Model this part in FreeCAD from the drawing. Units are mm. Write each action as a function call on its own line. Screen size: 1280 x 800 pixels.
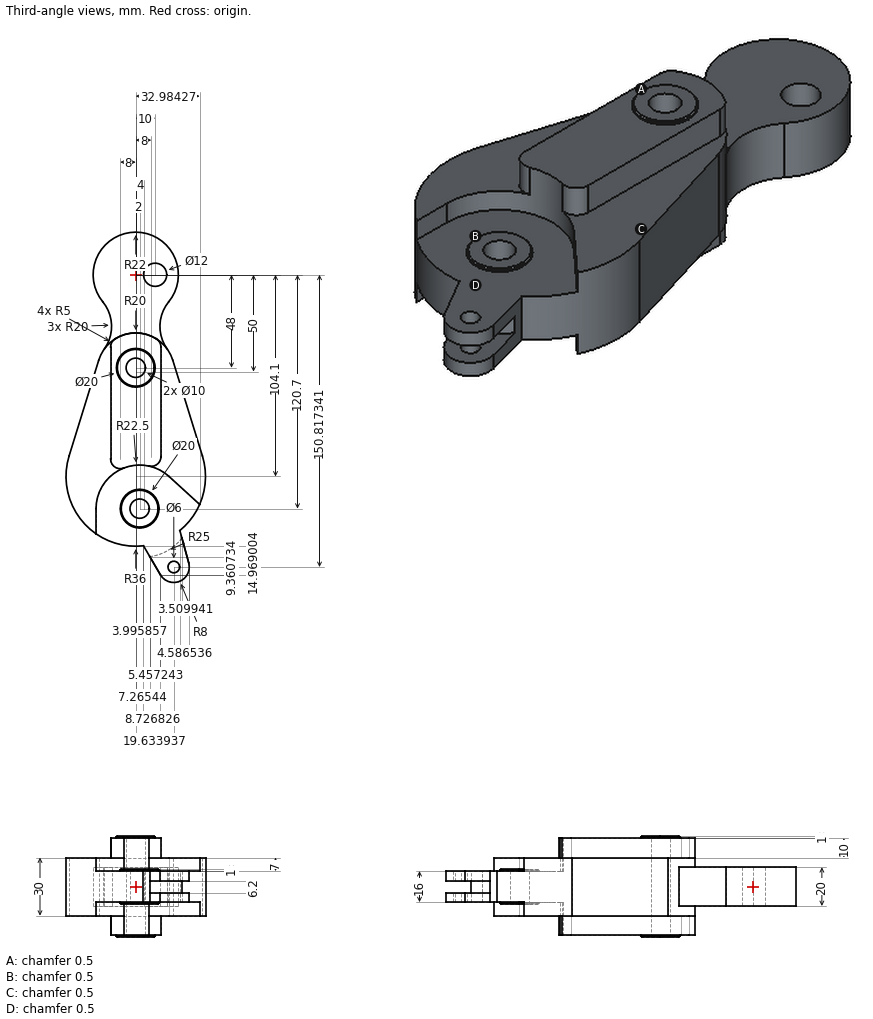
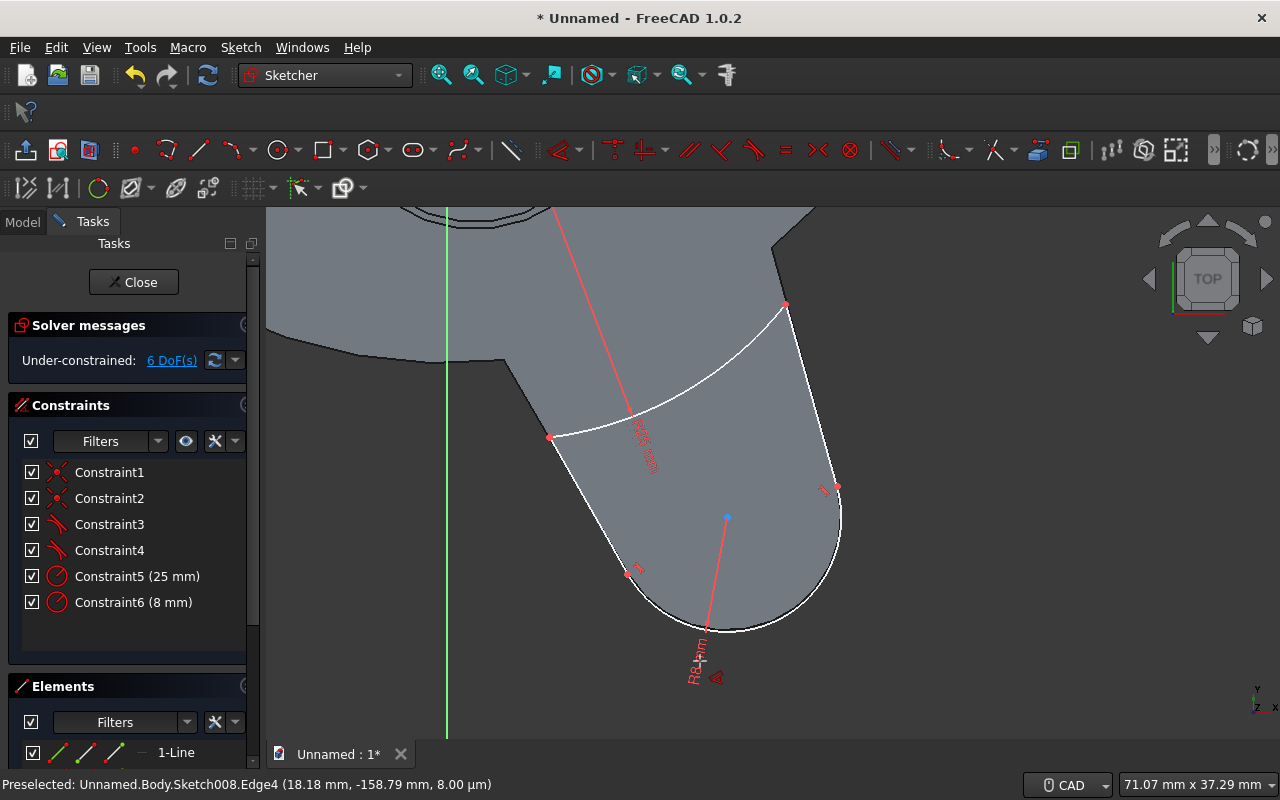
scroll(772, 711, down, 2)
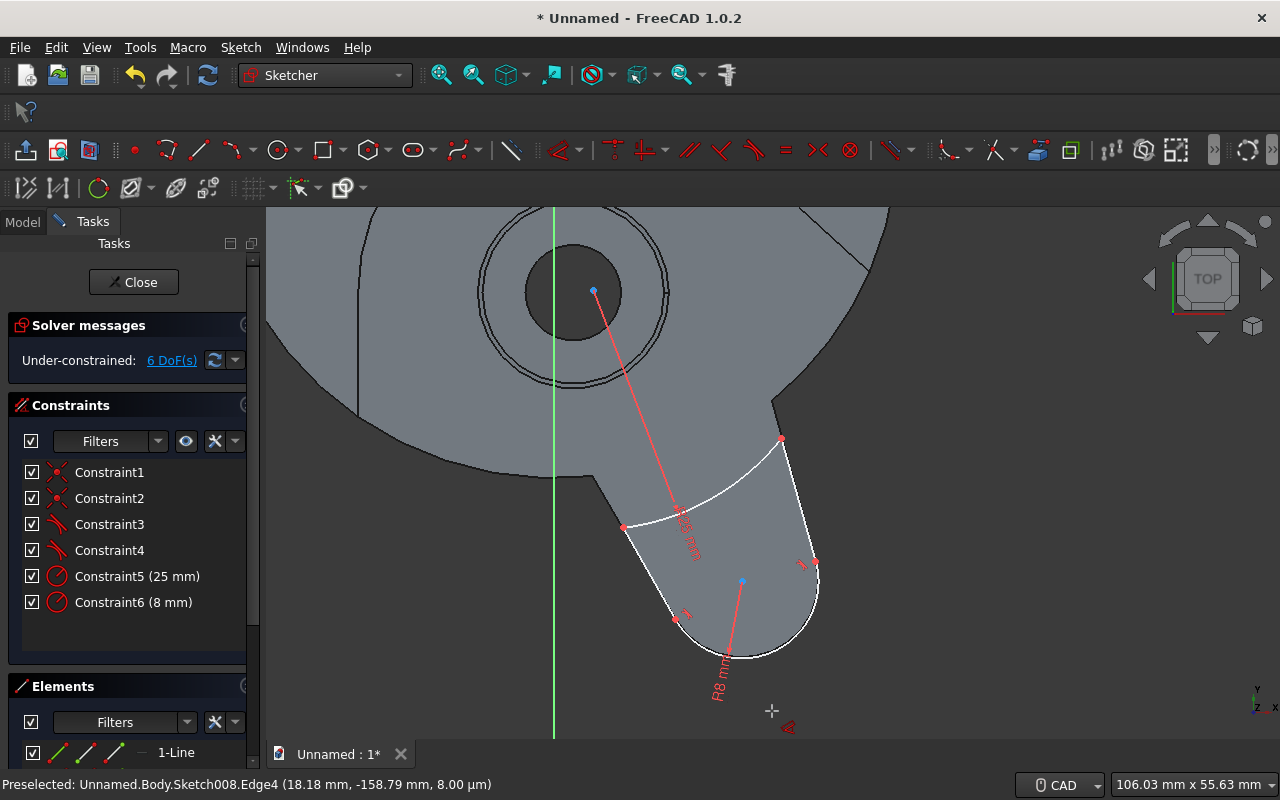
click(594, 291)
click(574, 325)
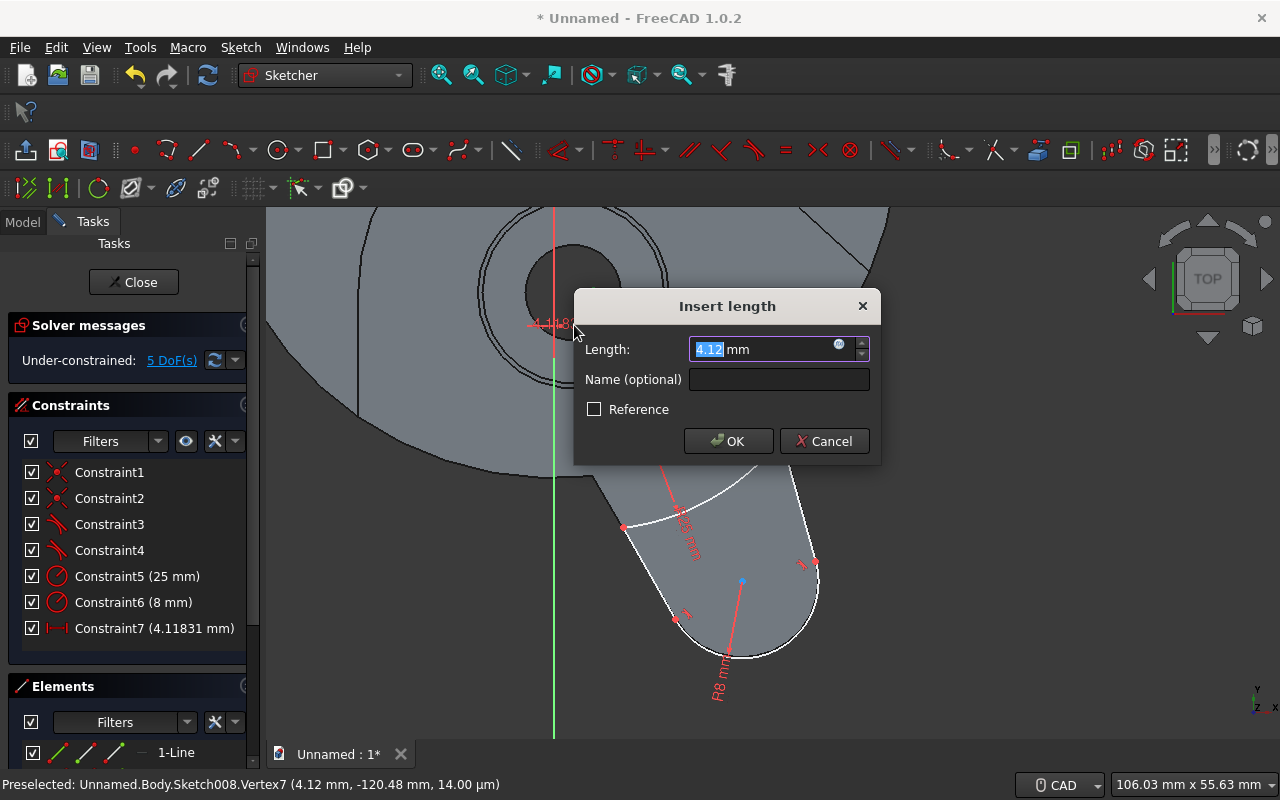
text(4)
key(Return)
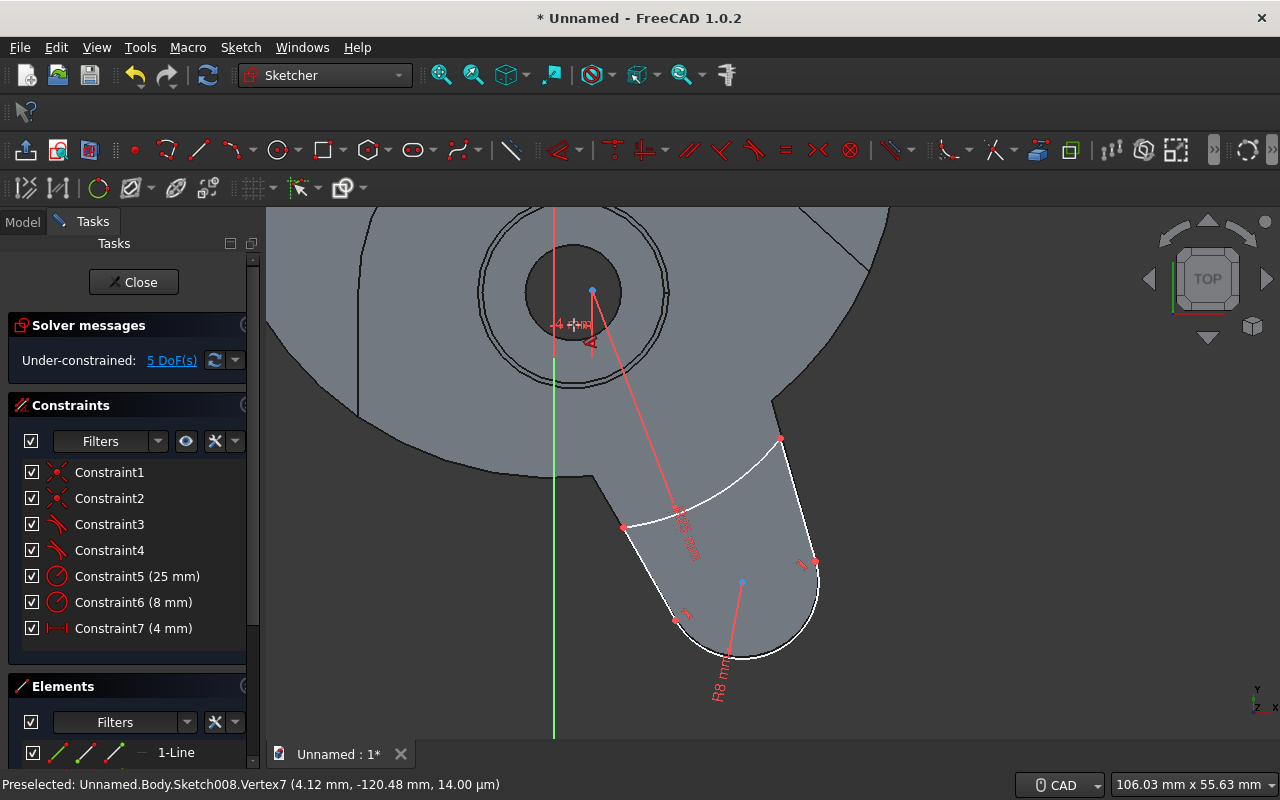
click(592, 291)
click(520, 263)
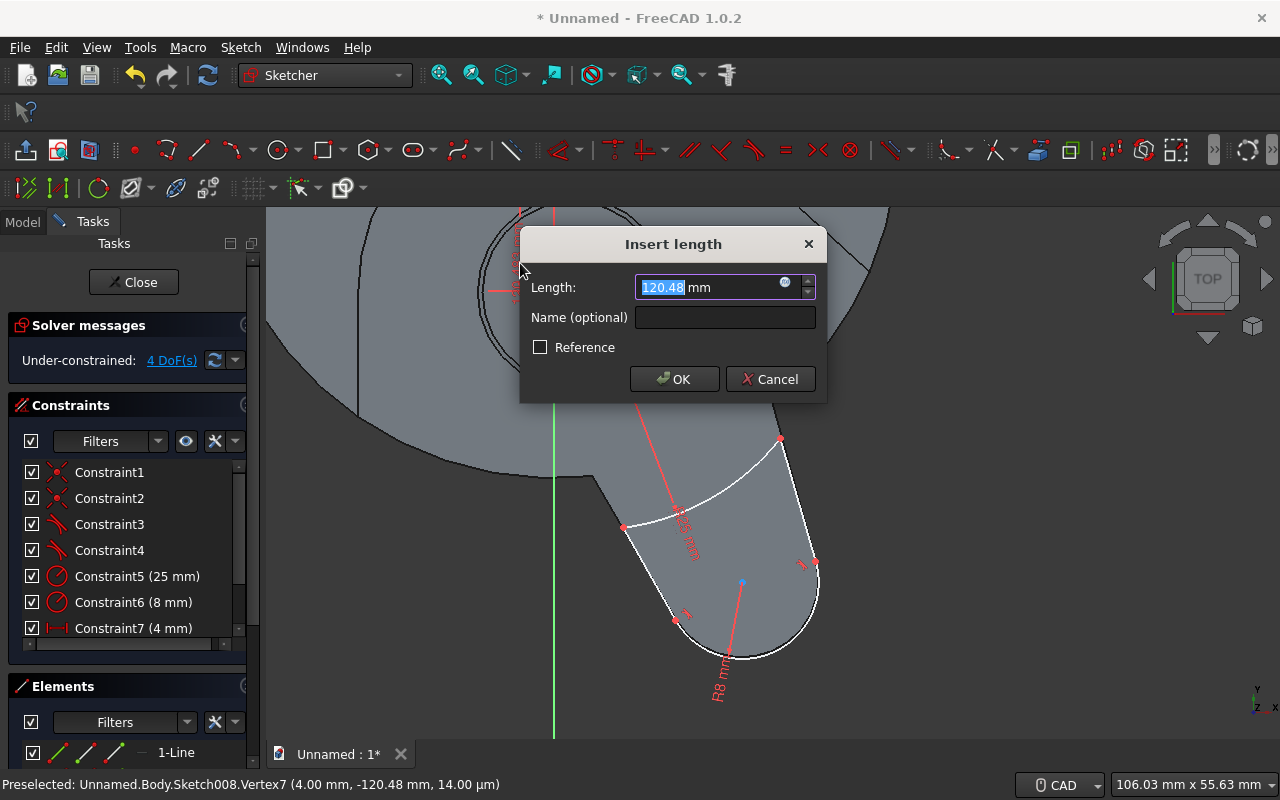
text(120.7)
key(Return)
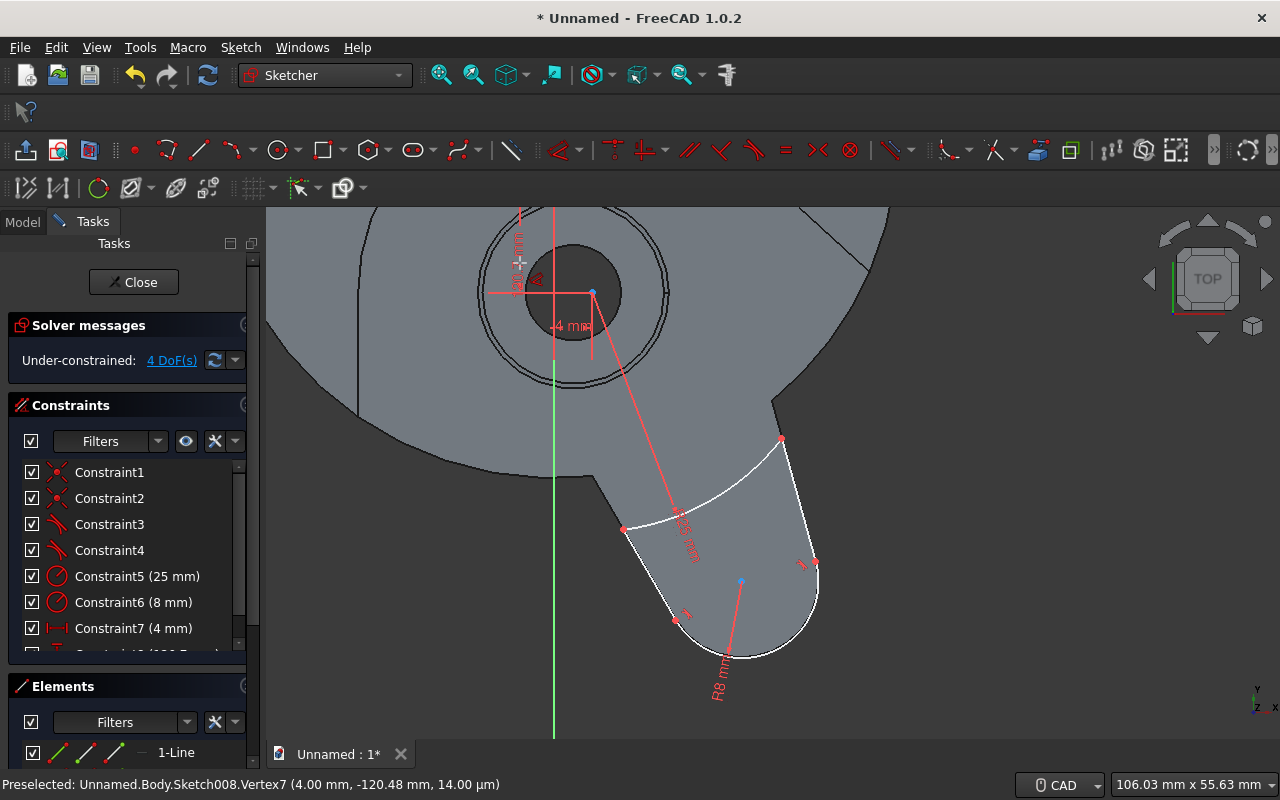
click(623, 530)
click(589, 564)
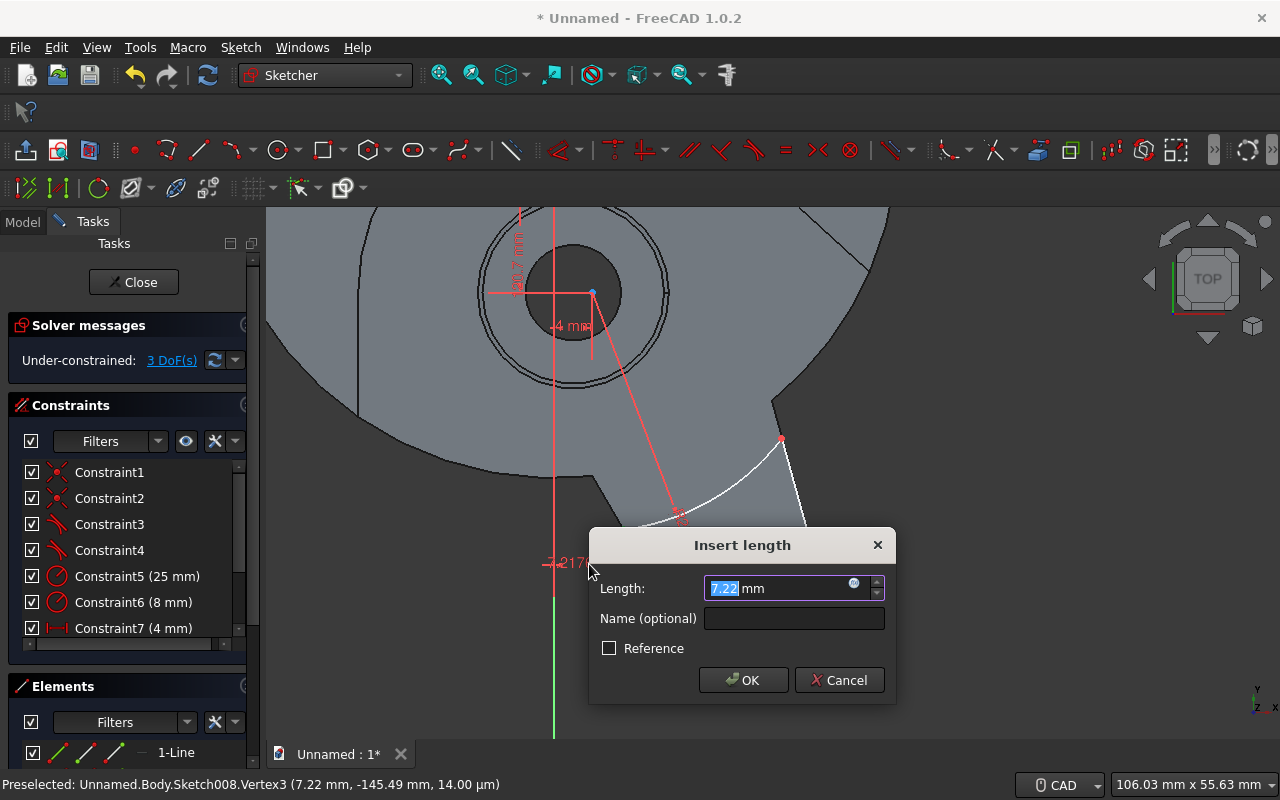
text(7.26544)
key(Return)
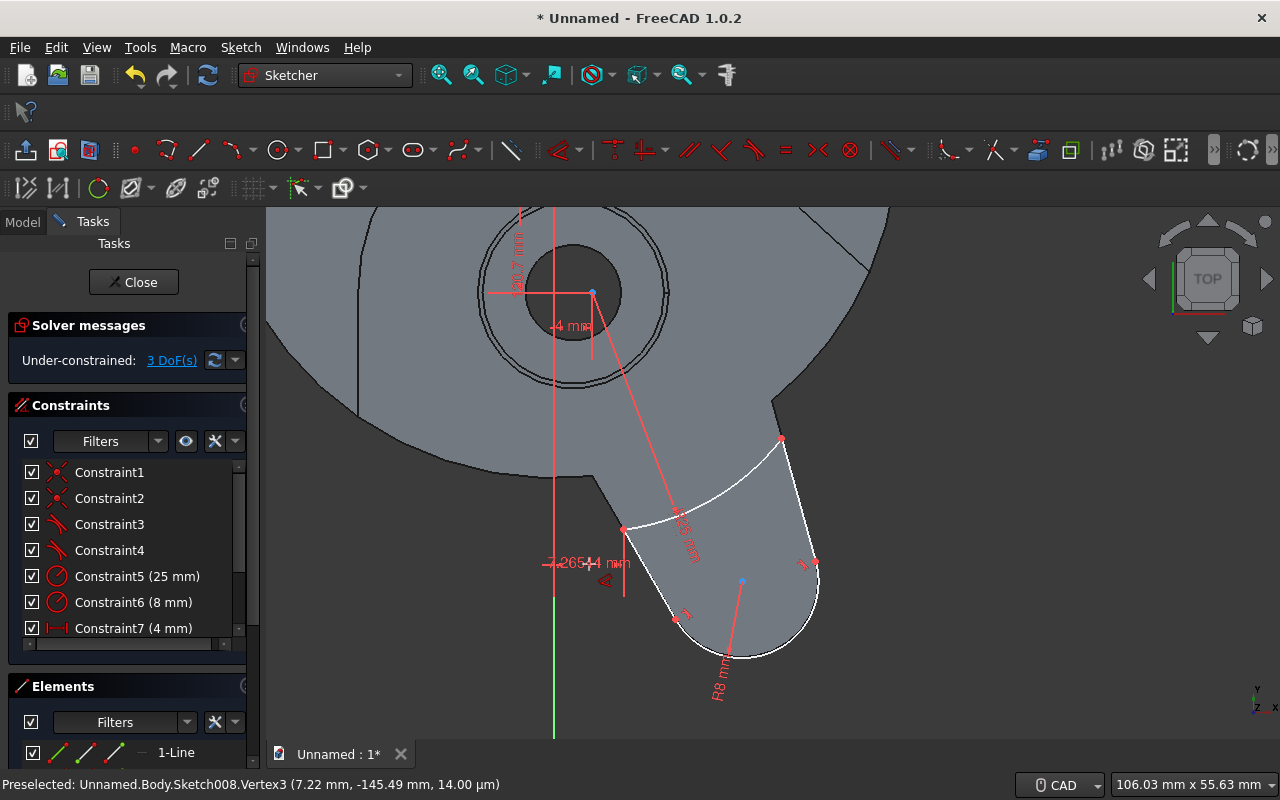
click(806, 524)
click(799, 405)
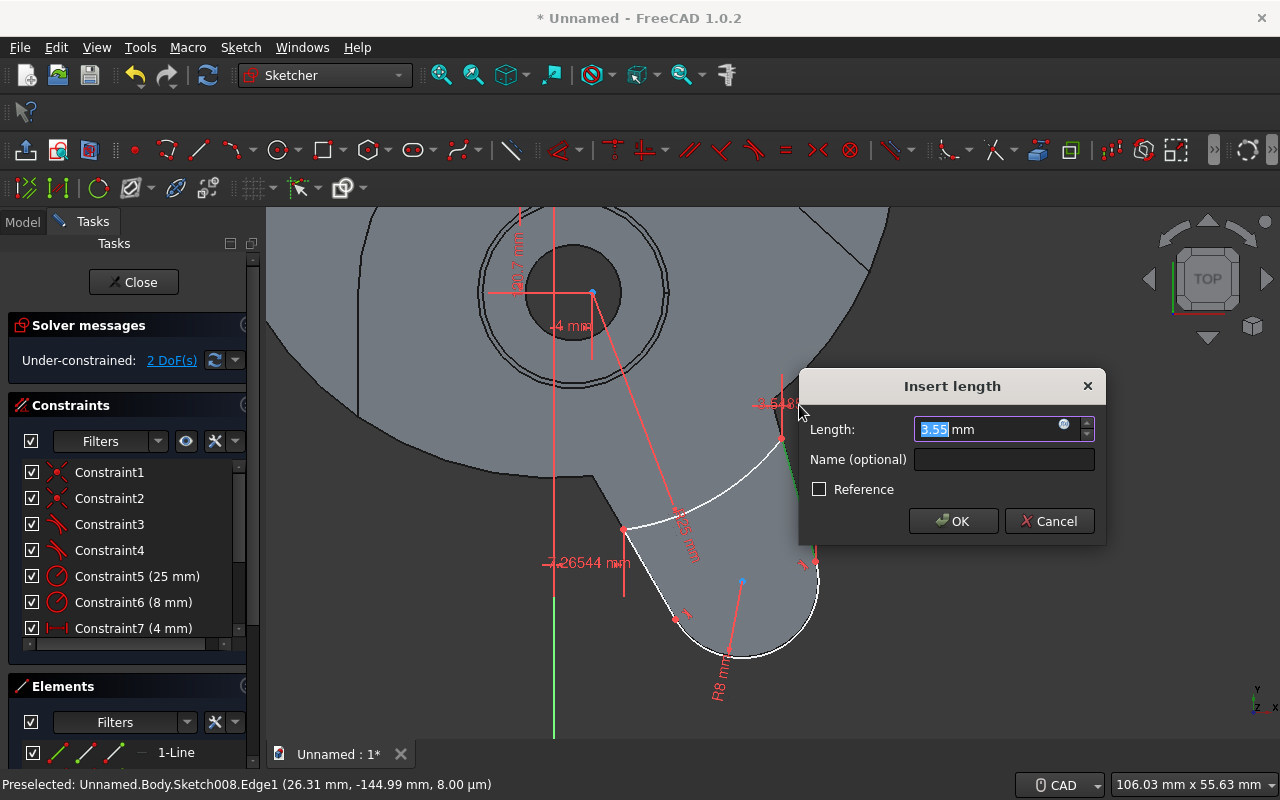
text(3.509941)
key(Return)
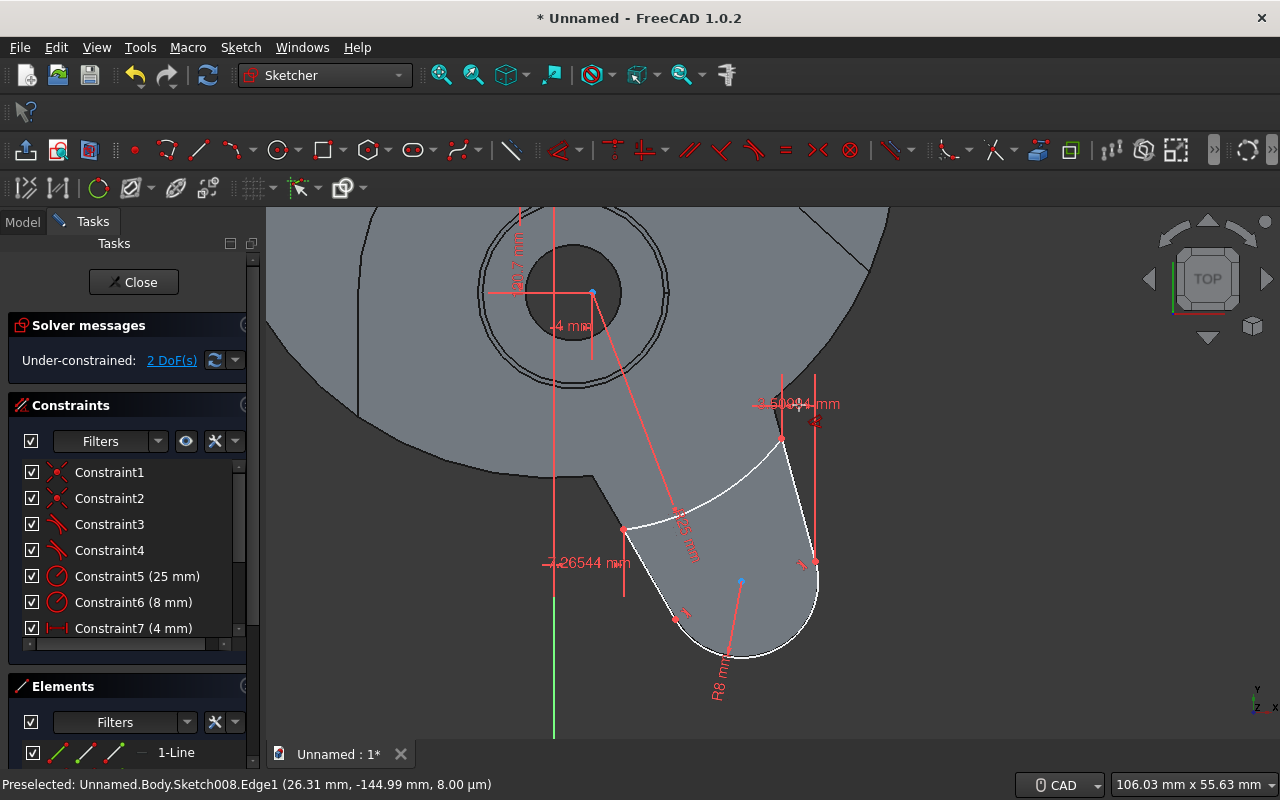
click(639, 557)
click(650, 654)